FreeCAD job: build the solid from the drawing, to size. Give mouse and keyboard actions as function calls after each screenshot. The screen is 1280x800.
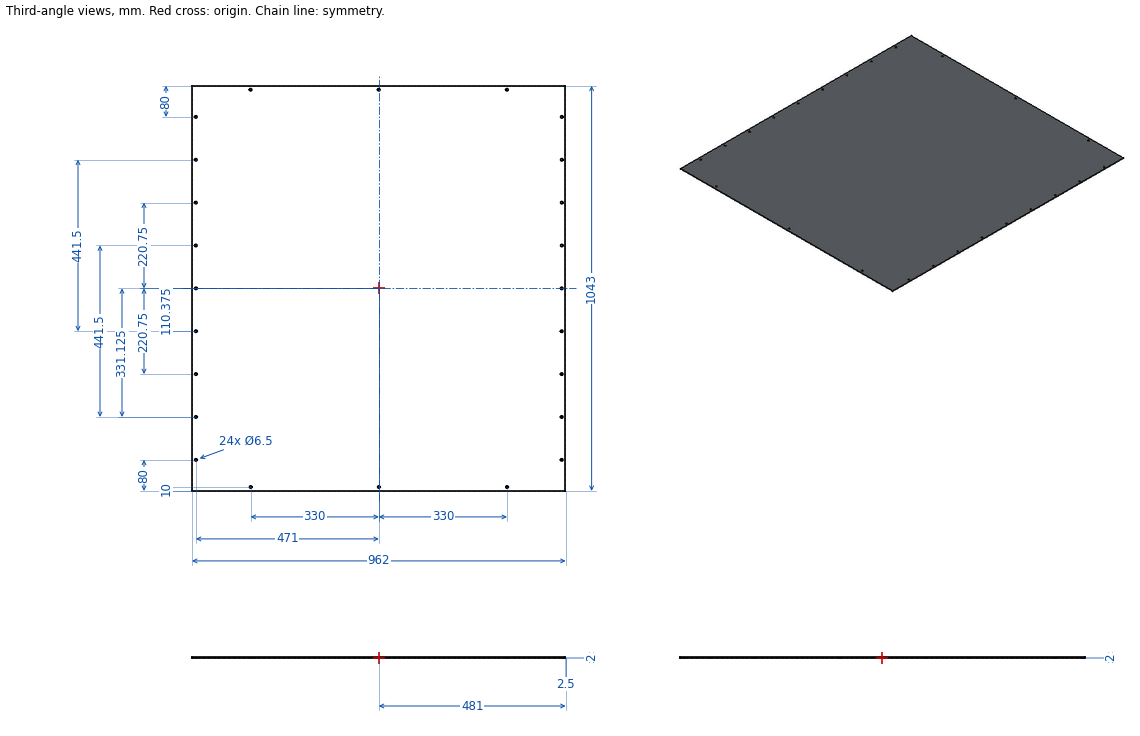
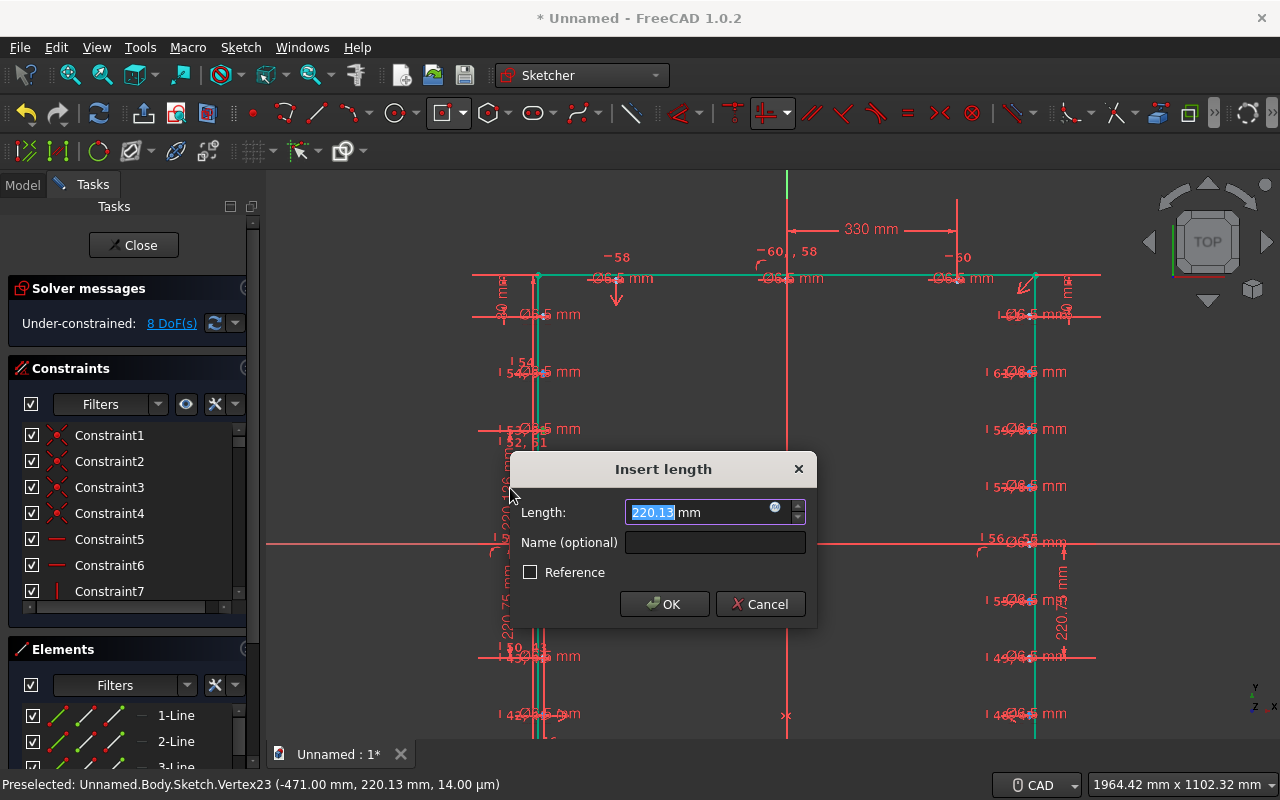
text(220.75)
key(Return)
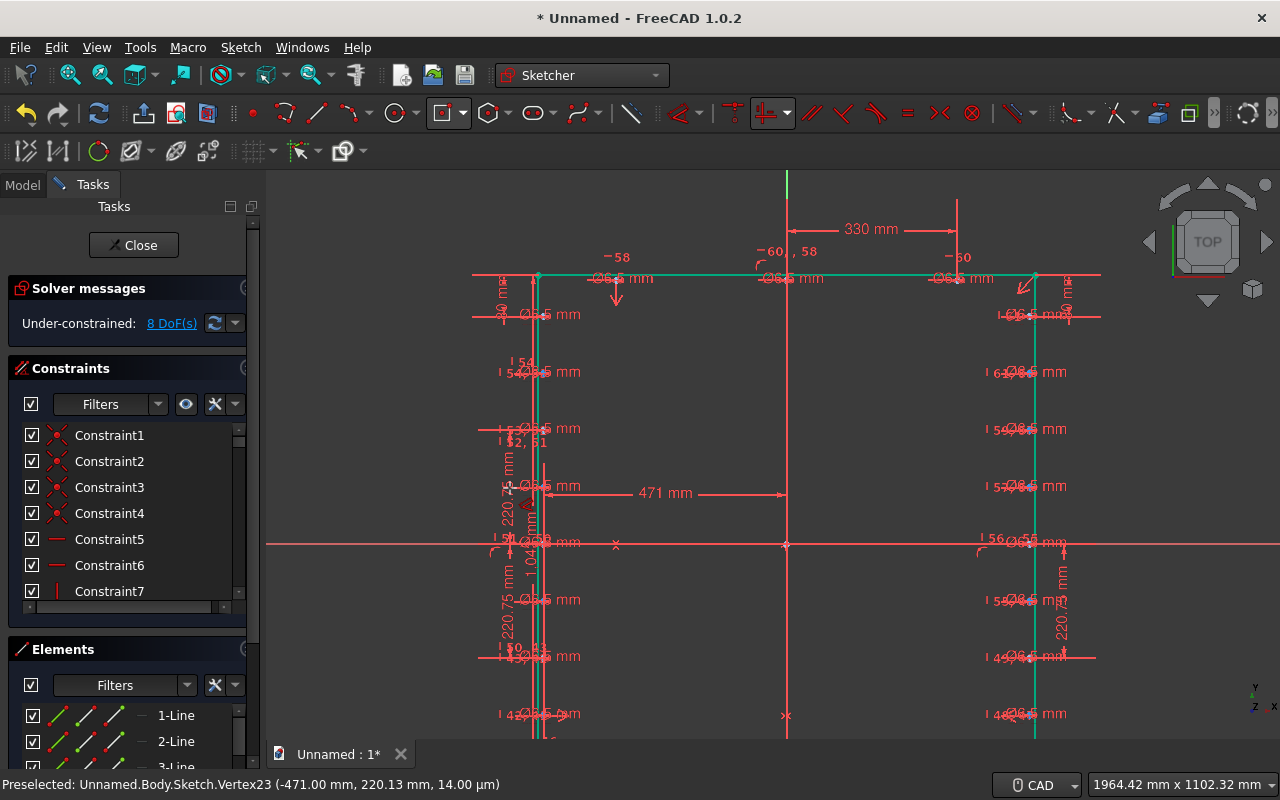
click(1030, 431)
click(1064, 488)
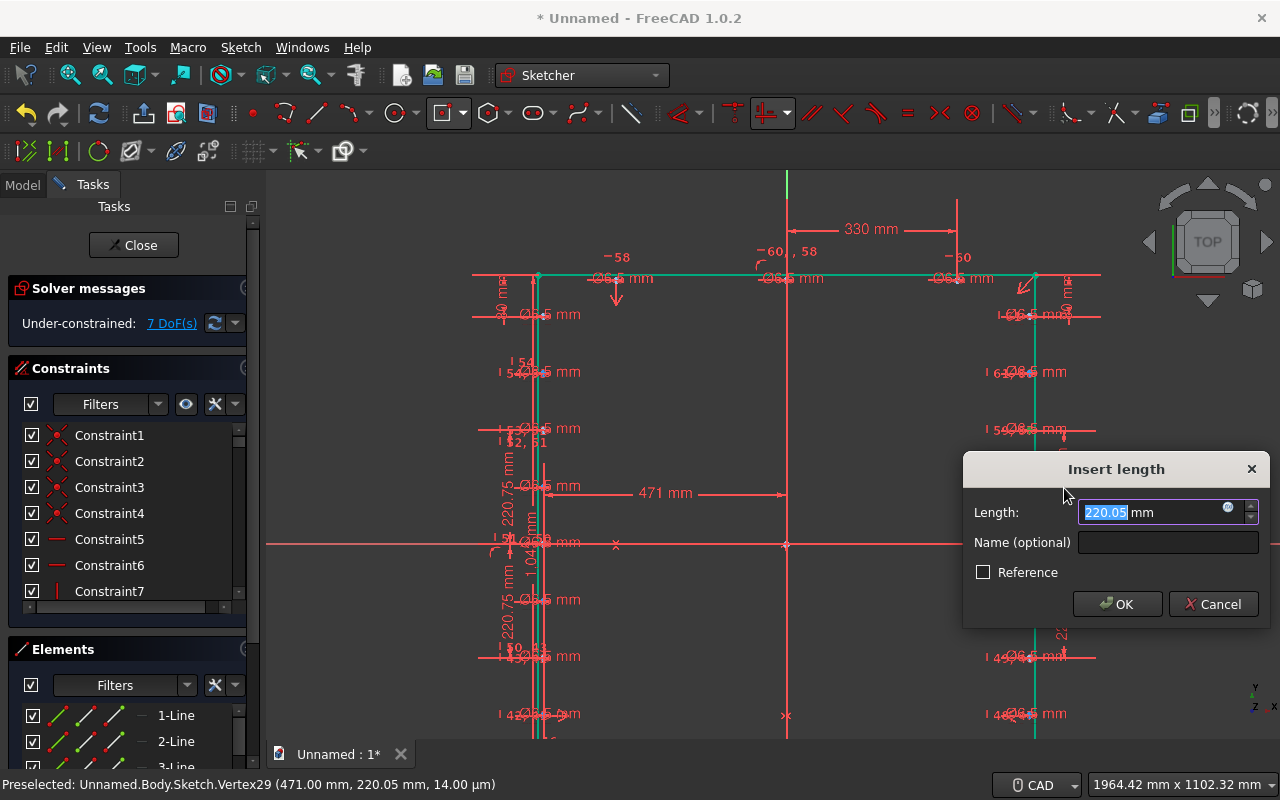
text(220.75)
key(Return)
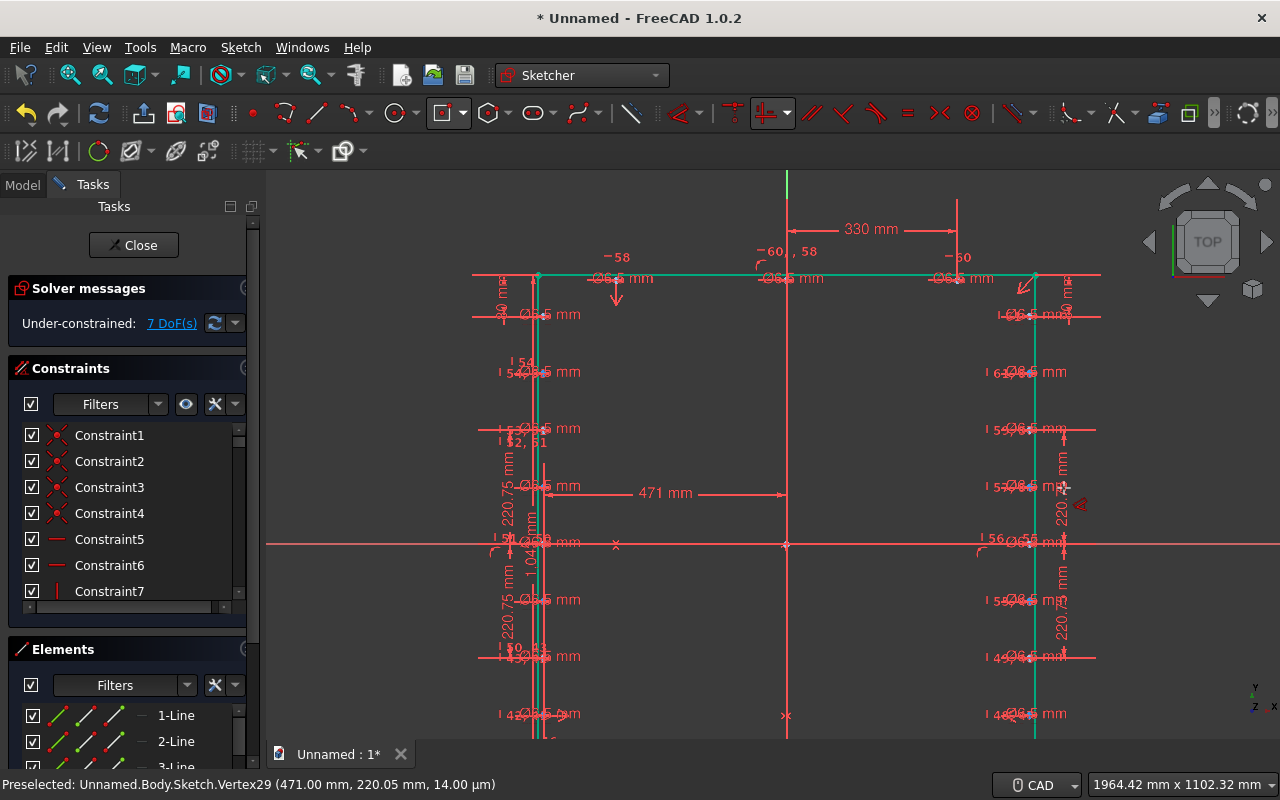
scroll(537, 272, down, 2)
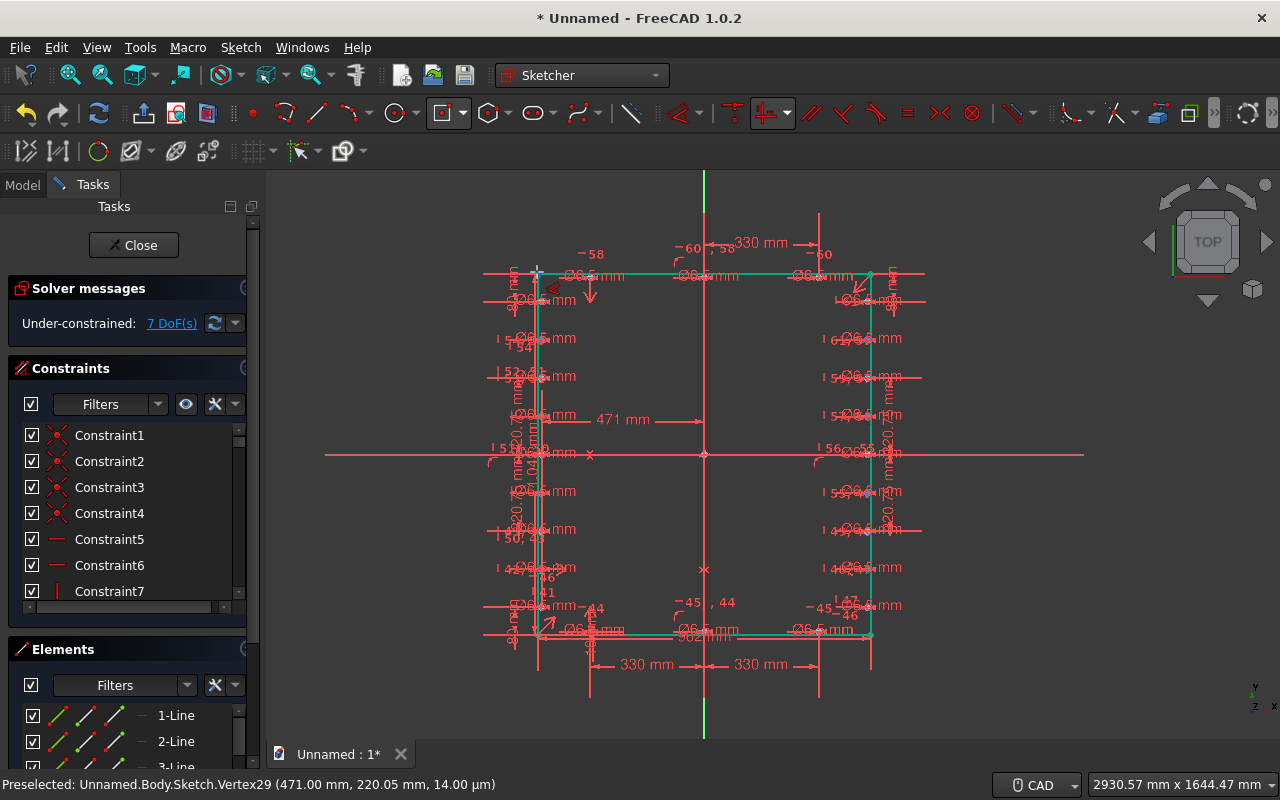
click(542, 569)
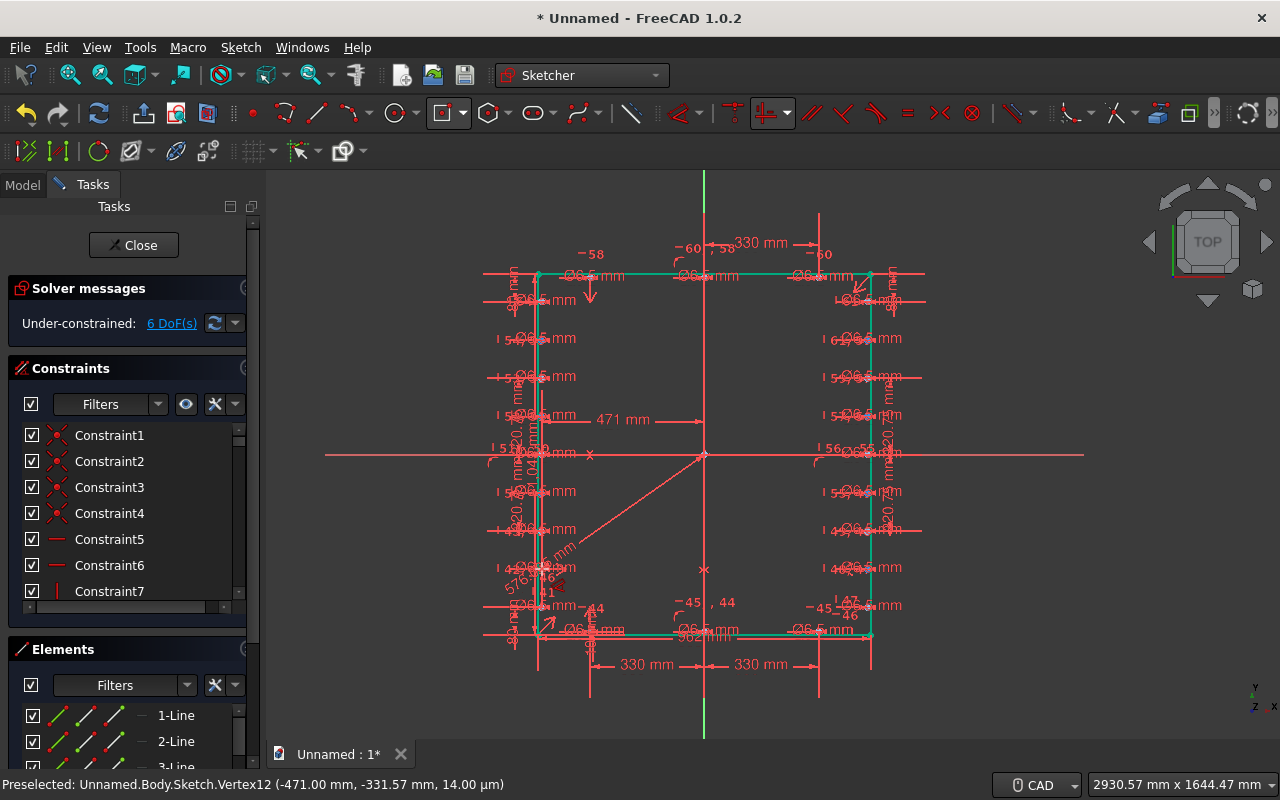
click(542, 417)
click(508, 528)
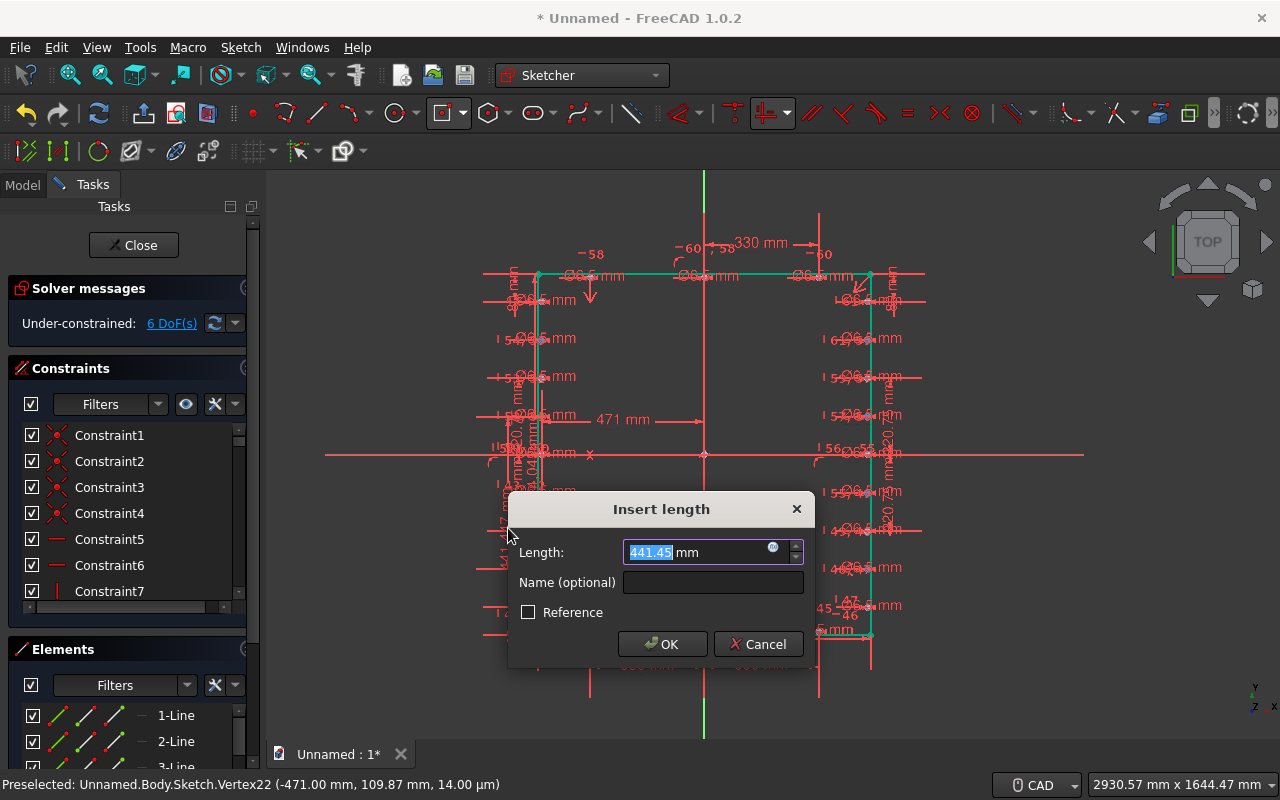
text(441.5)
key(Return)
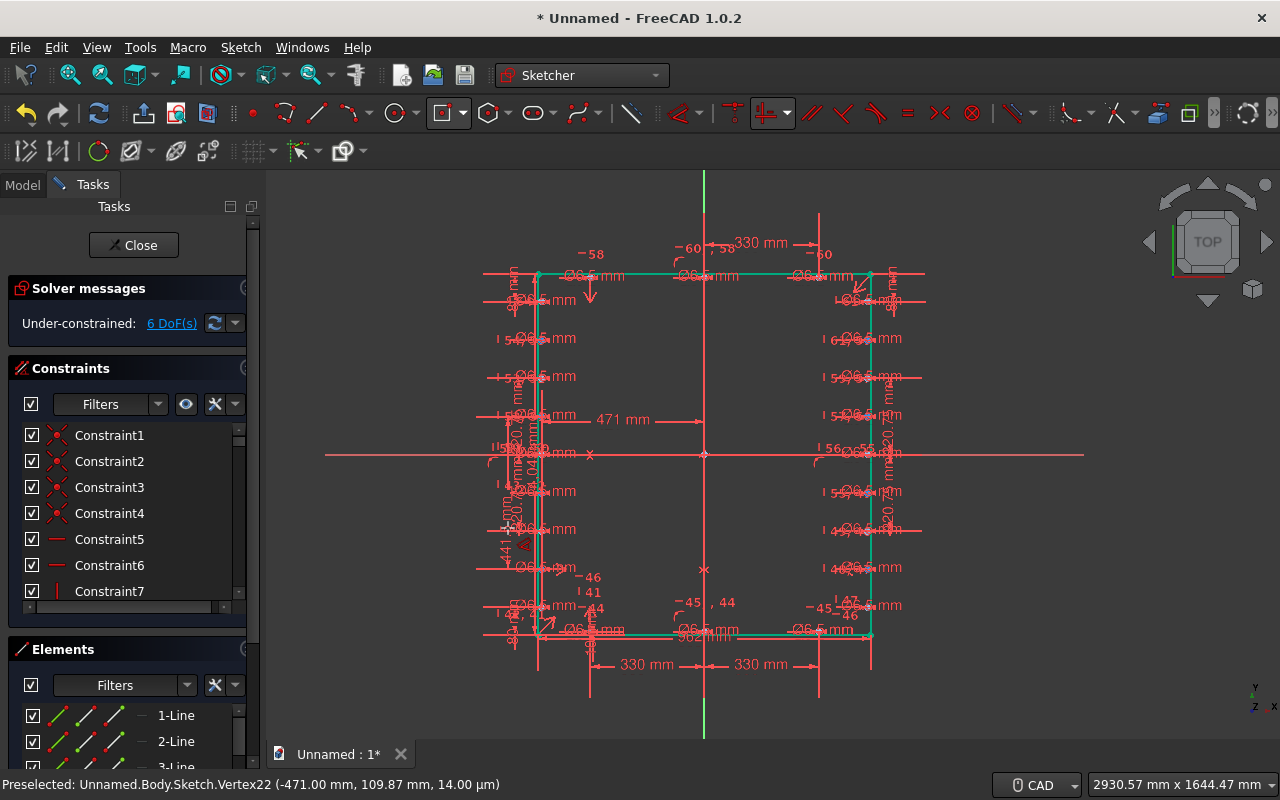
click(542, 493)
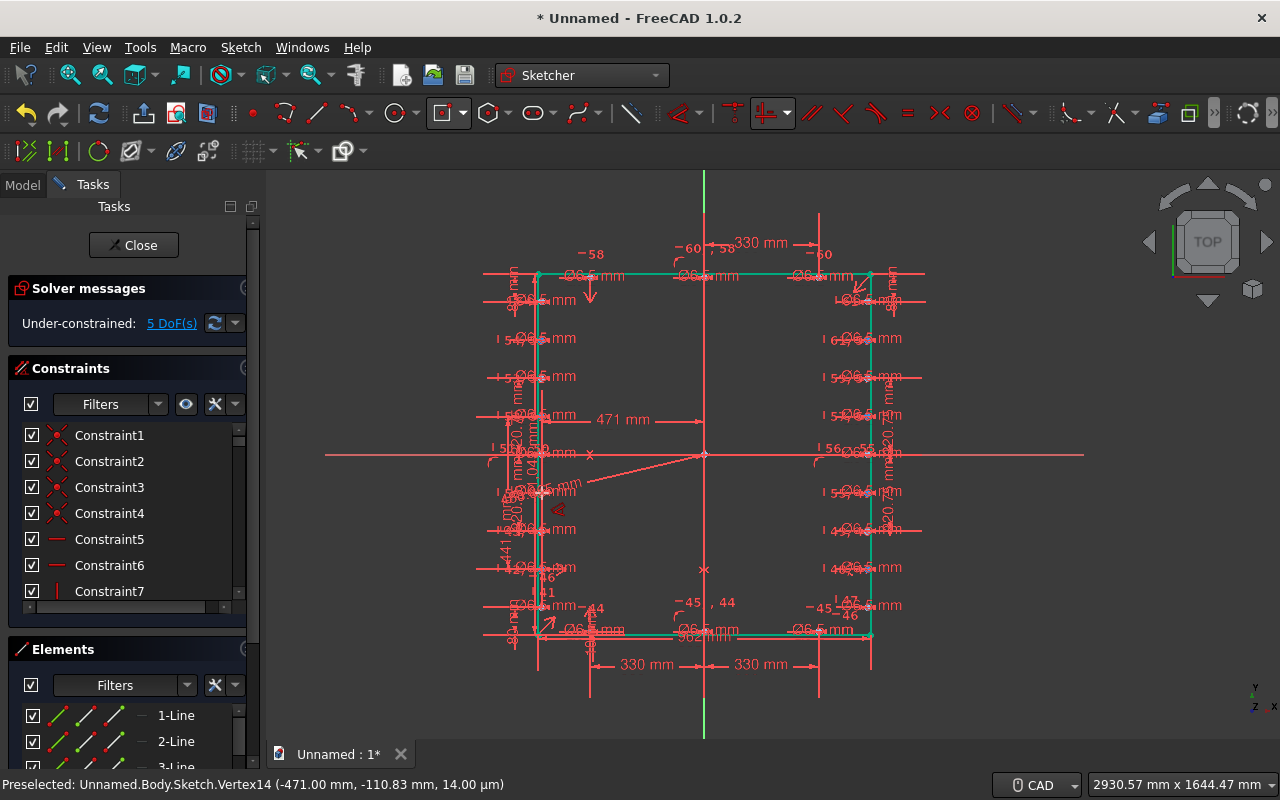
click(542, 340)
click(508, 381)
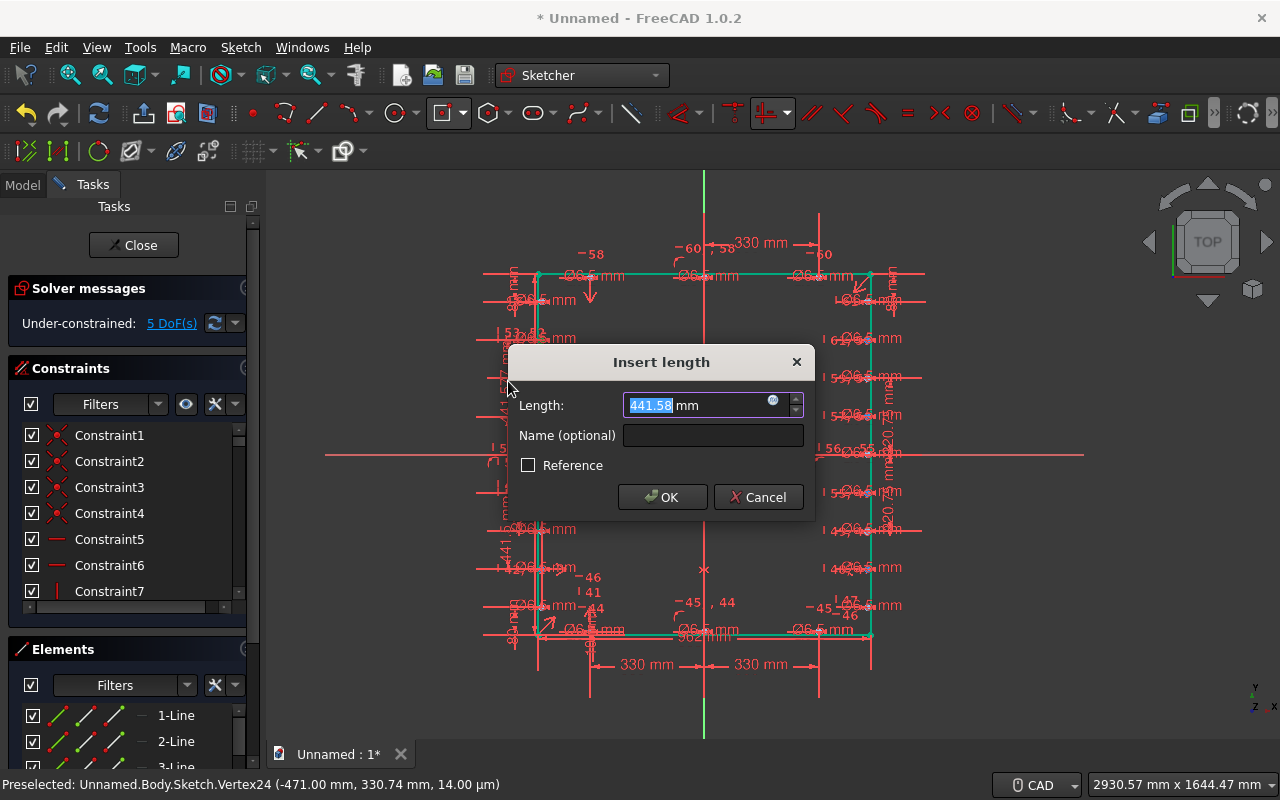
text(441.5)
key(Return)